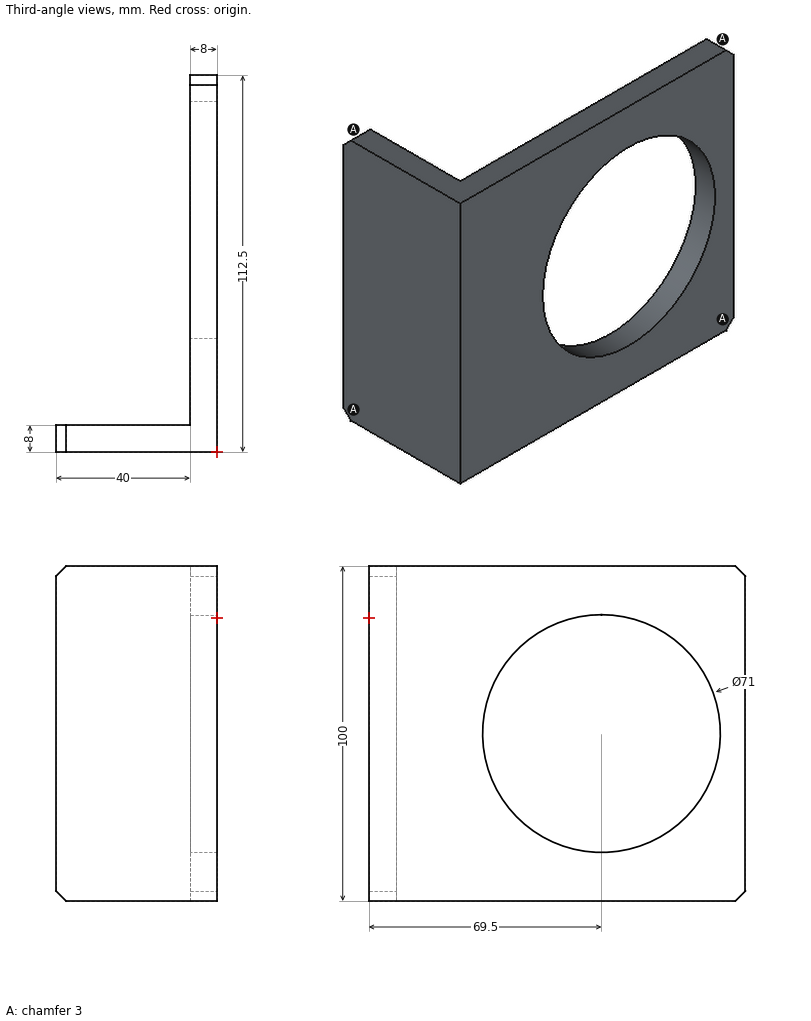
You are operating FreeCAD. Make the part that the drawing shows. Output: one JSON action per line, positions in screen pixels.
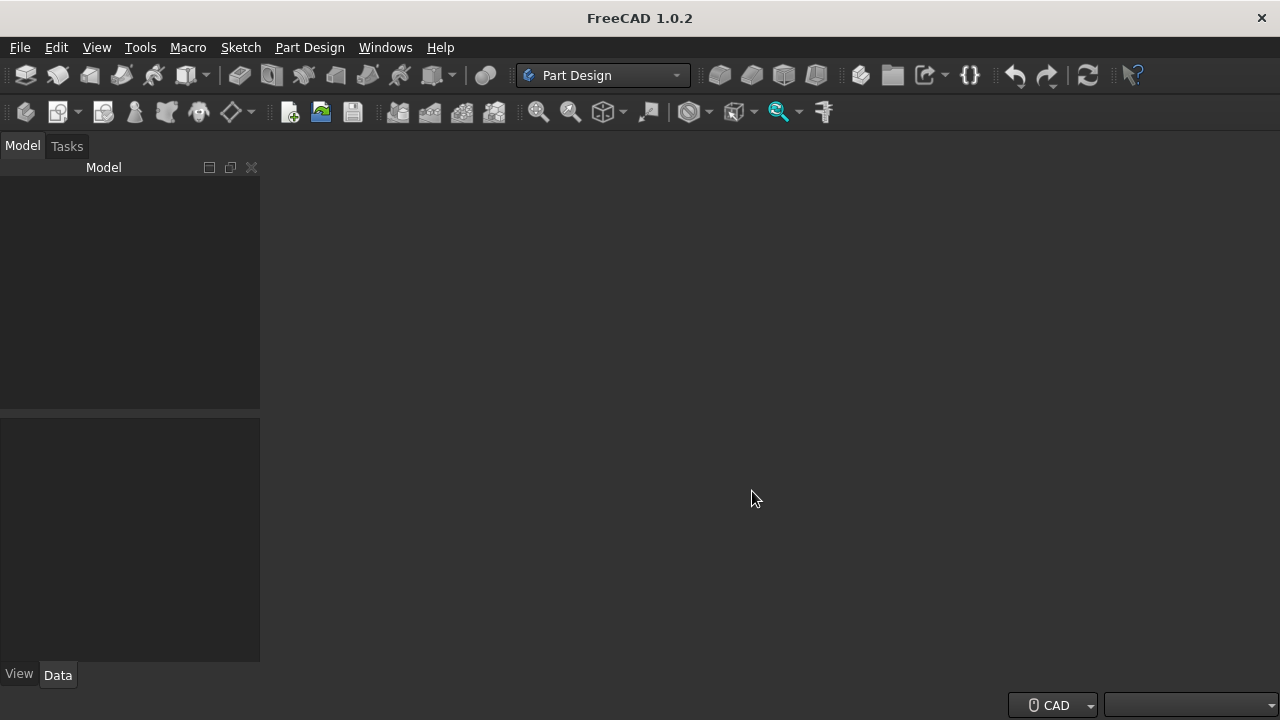
{"action": "left_click", "coordinate": [290, 112]}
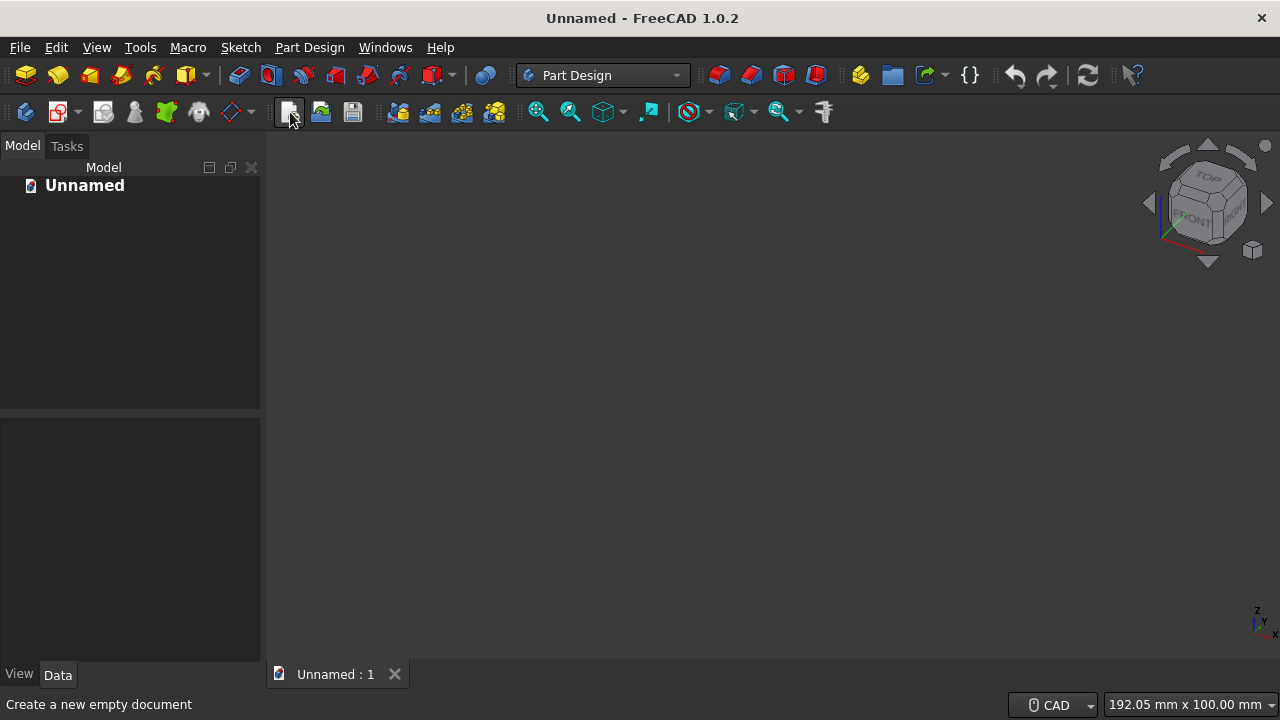
{"action": "left_click", "coordinate": [26, 112]}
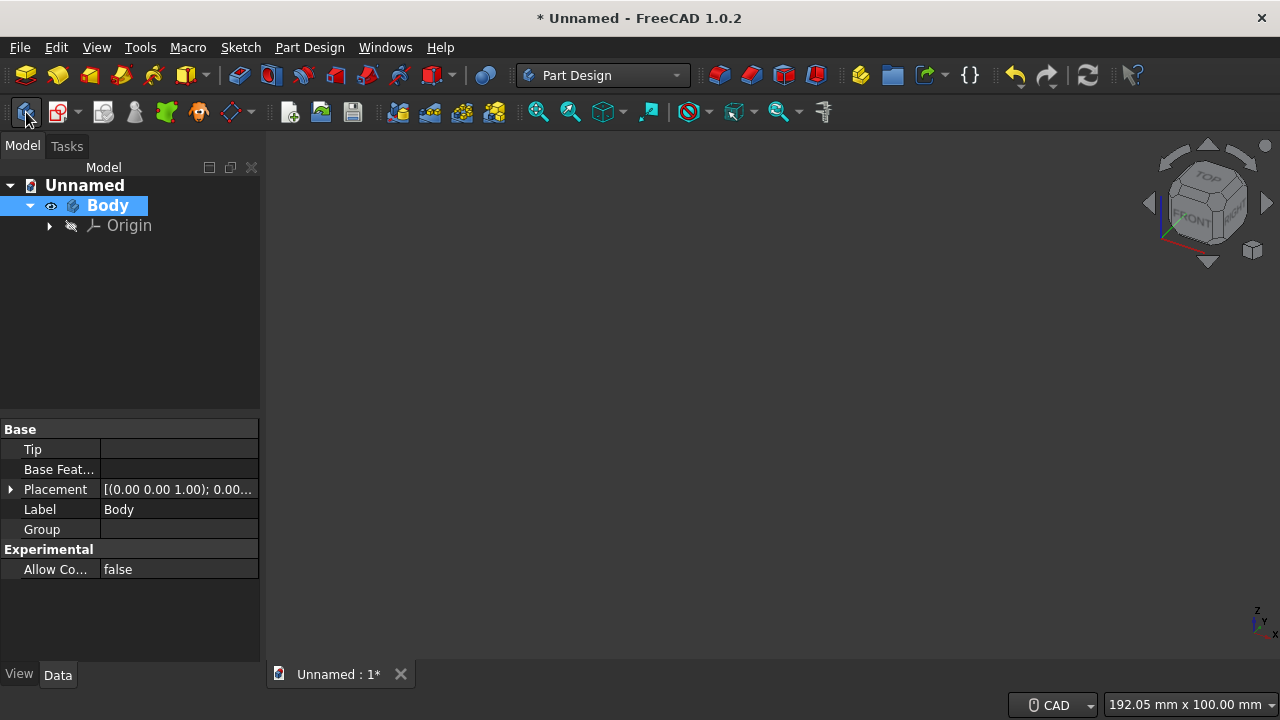
{"action": "left_click", "coordinate": [50, 226]}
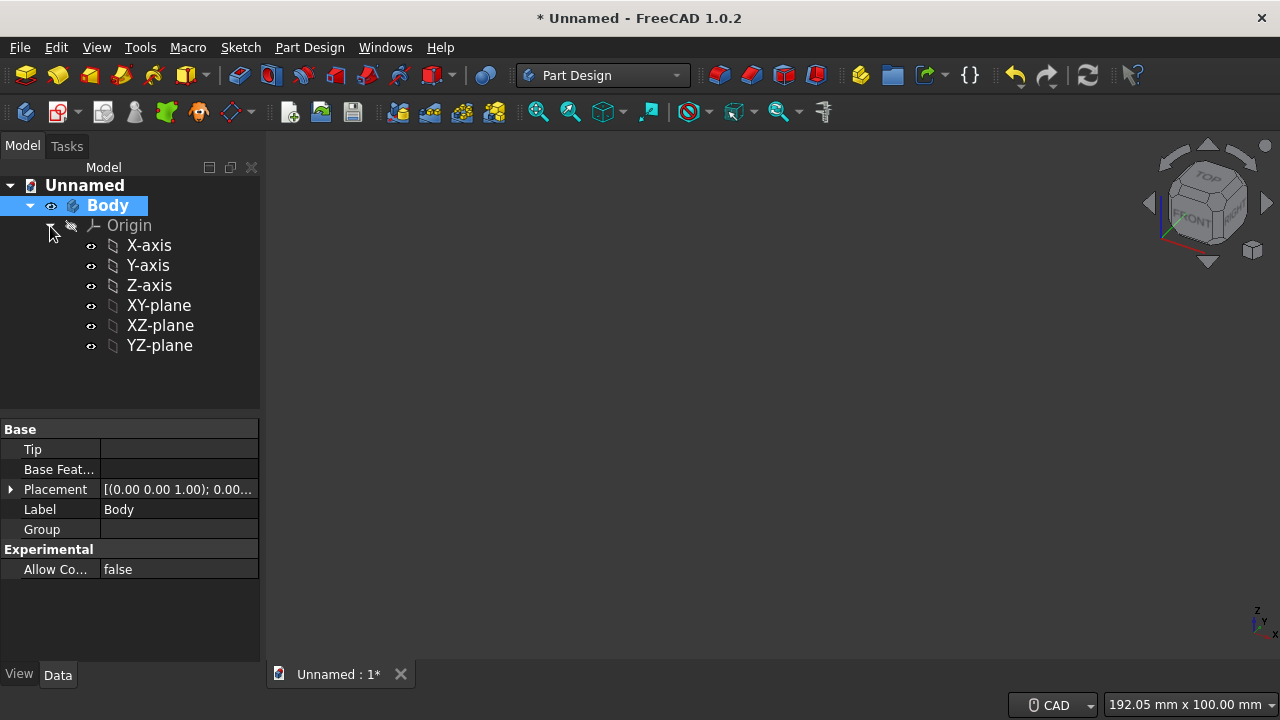
{"action": "left_click", "coordinate": [136, 306]}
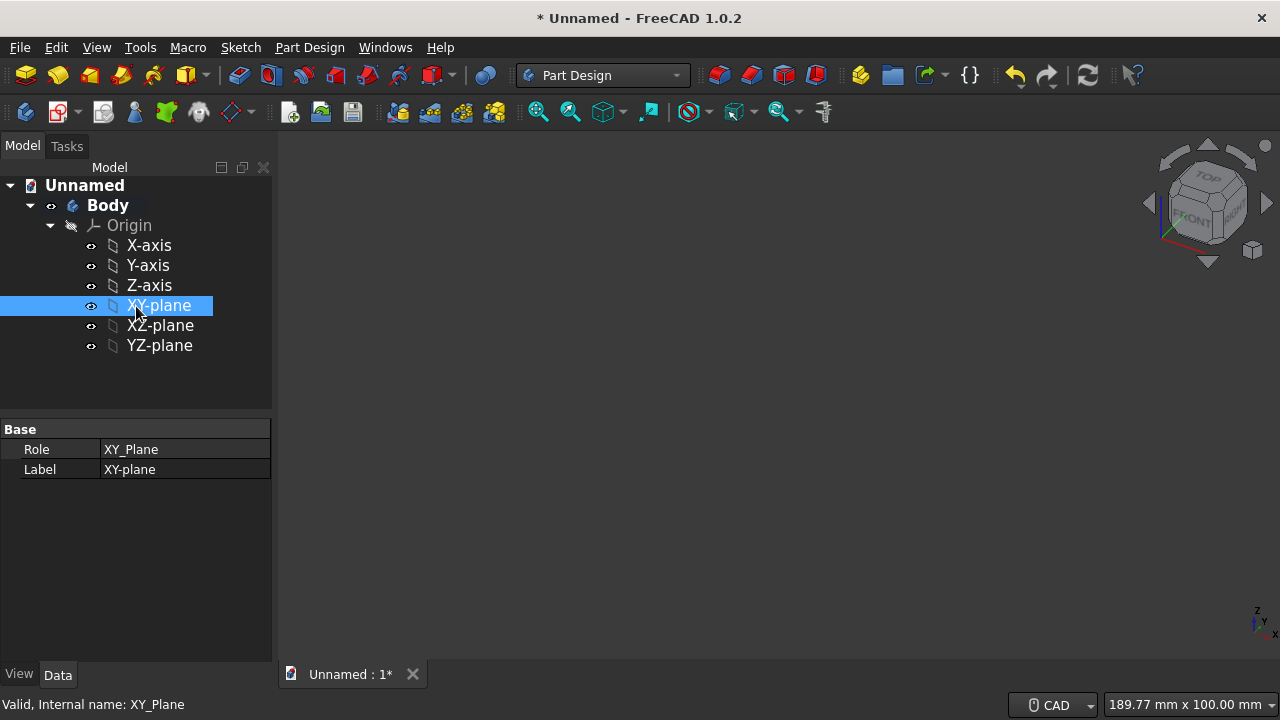
{"action": "left_click", "coordinate": [232, 112]}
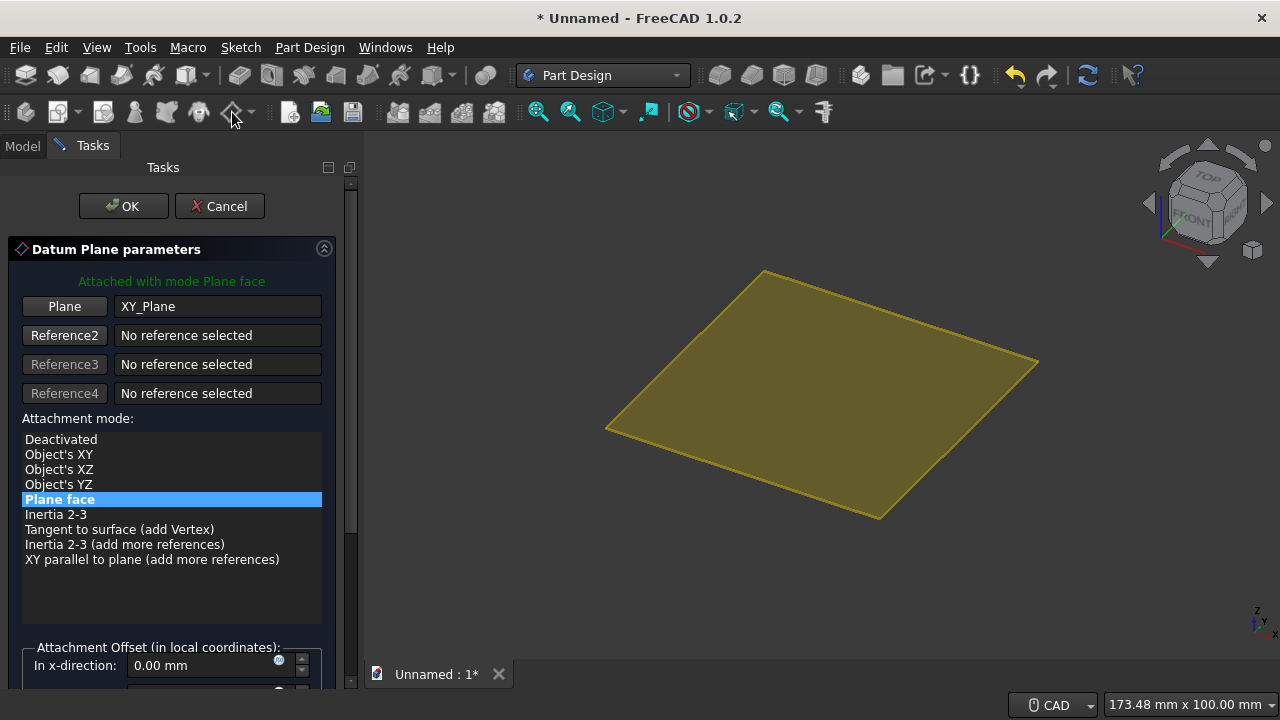
{"action": "scroll", "coordinate": [351, 432], "scroll_direction": "down", "scroll_amount": 2}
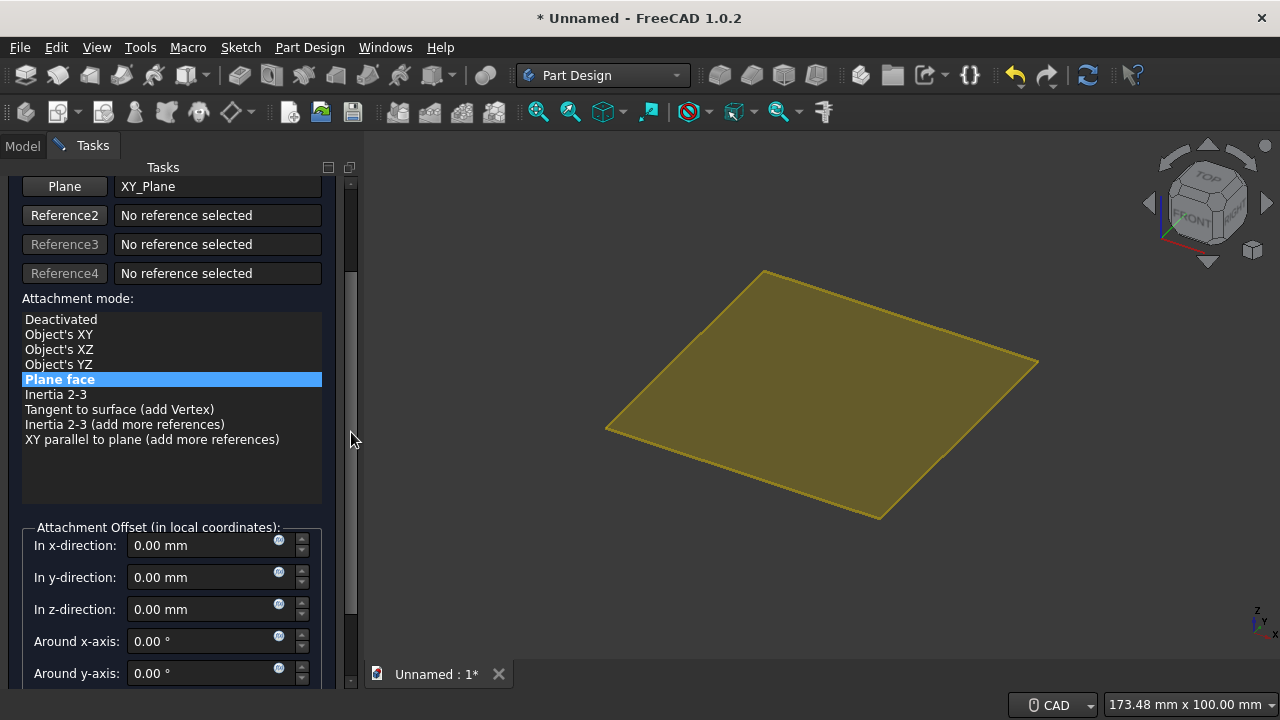
{"action": "triple_click", "coordinate": [210, 609]}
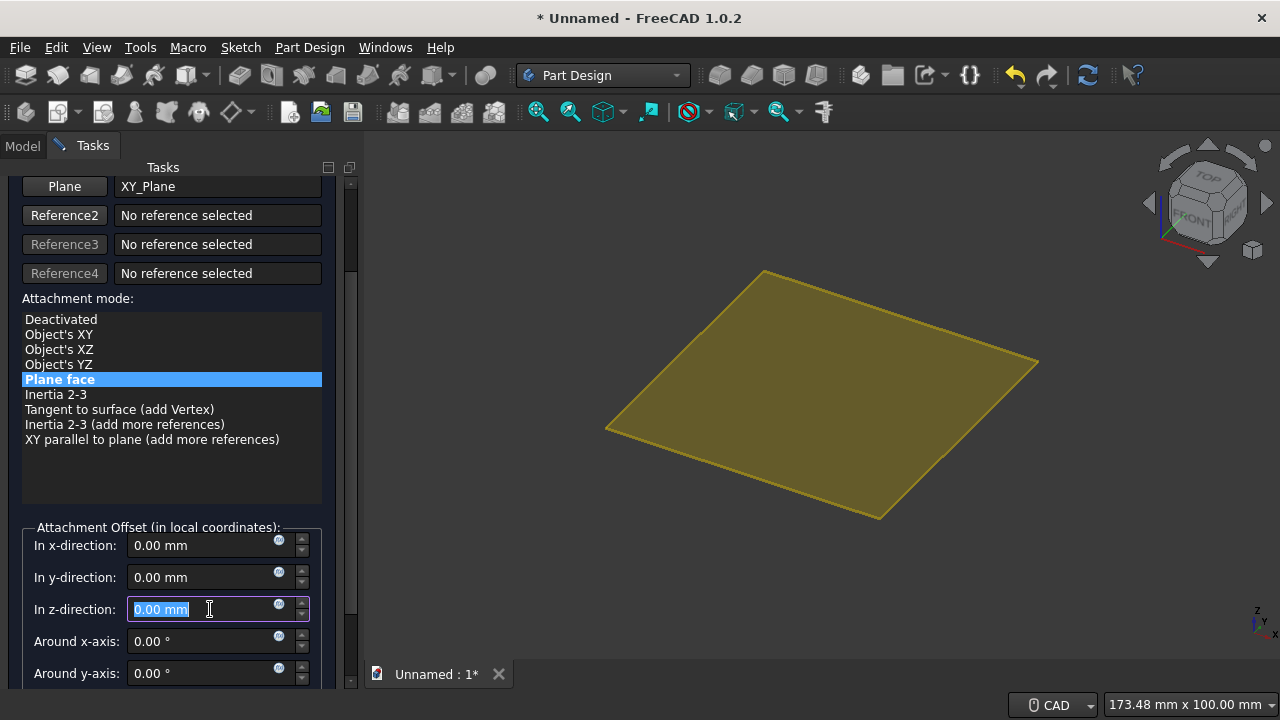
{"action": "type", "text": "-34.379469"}
{"action": "key", "text": "Tab"}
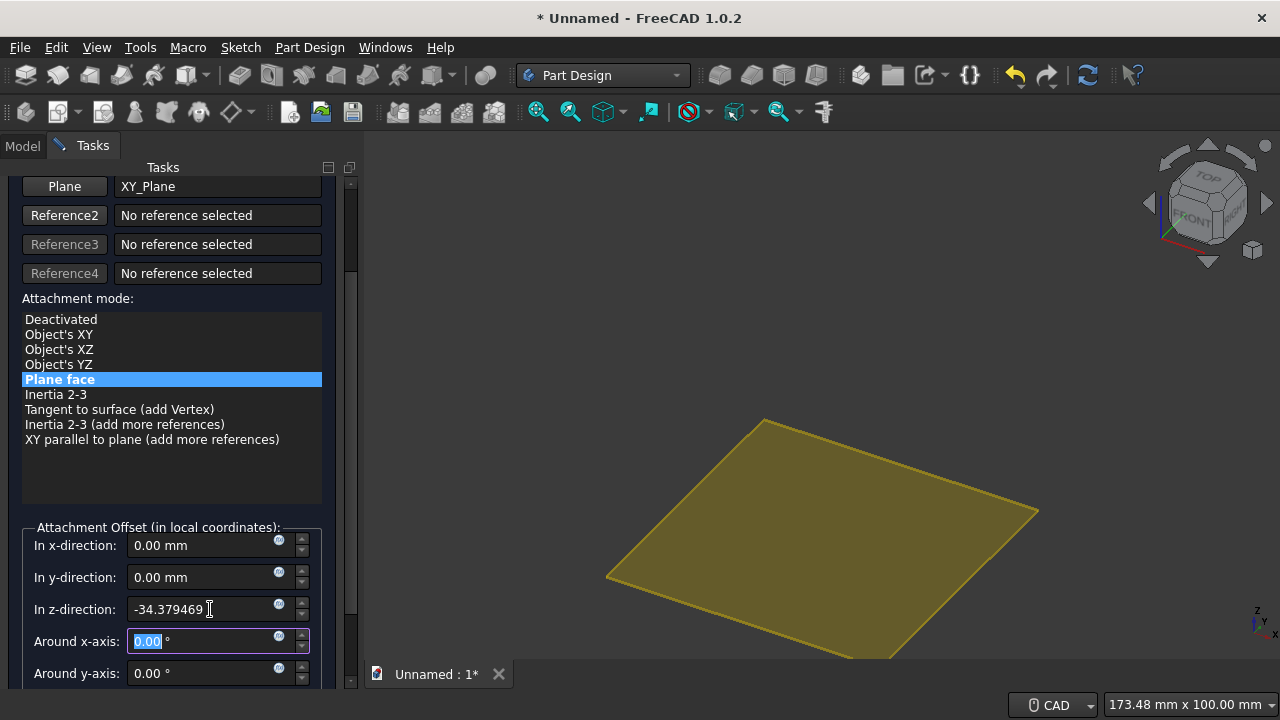
{"action": "scroll", "coordinate": [351, 432], "scroll_direction": "up", "scroll_amount": 3}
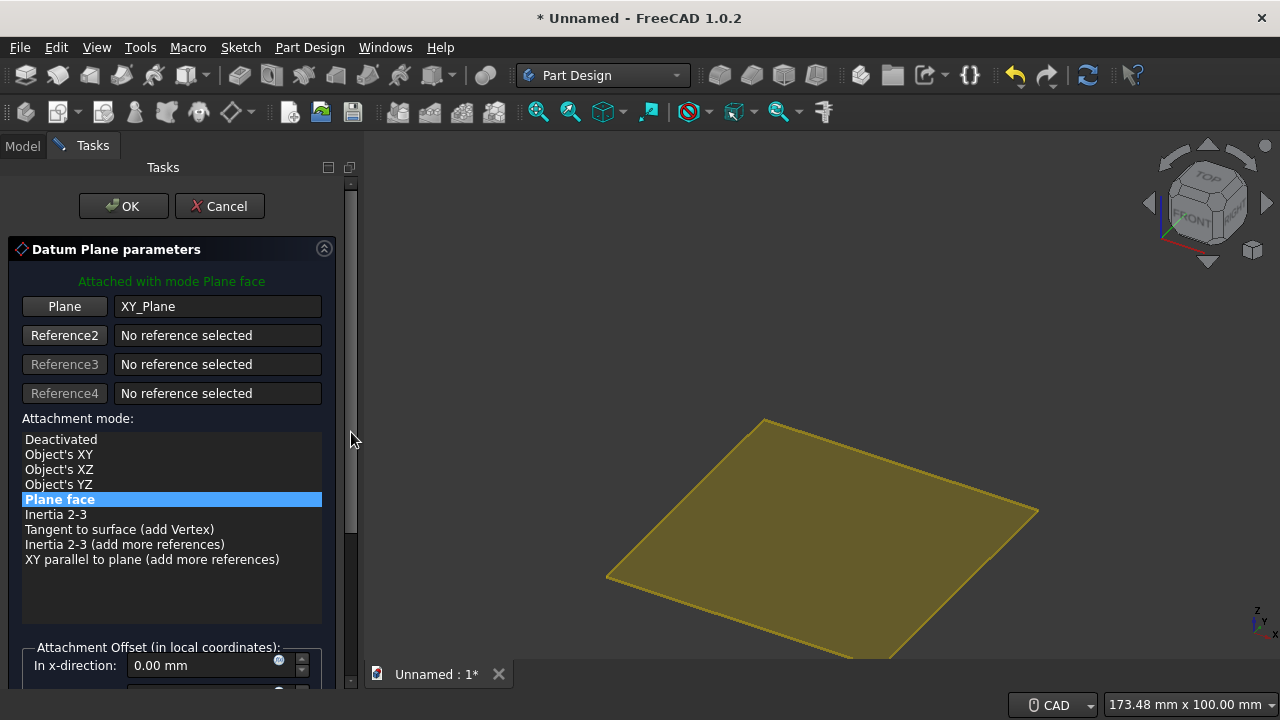
{"action": "left_click", "coordinate": [124, 206]}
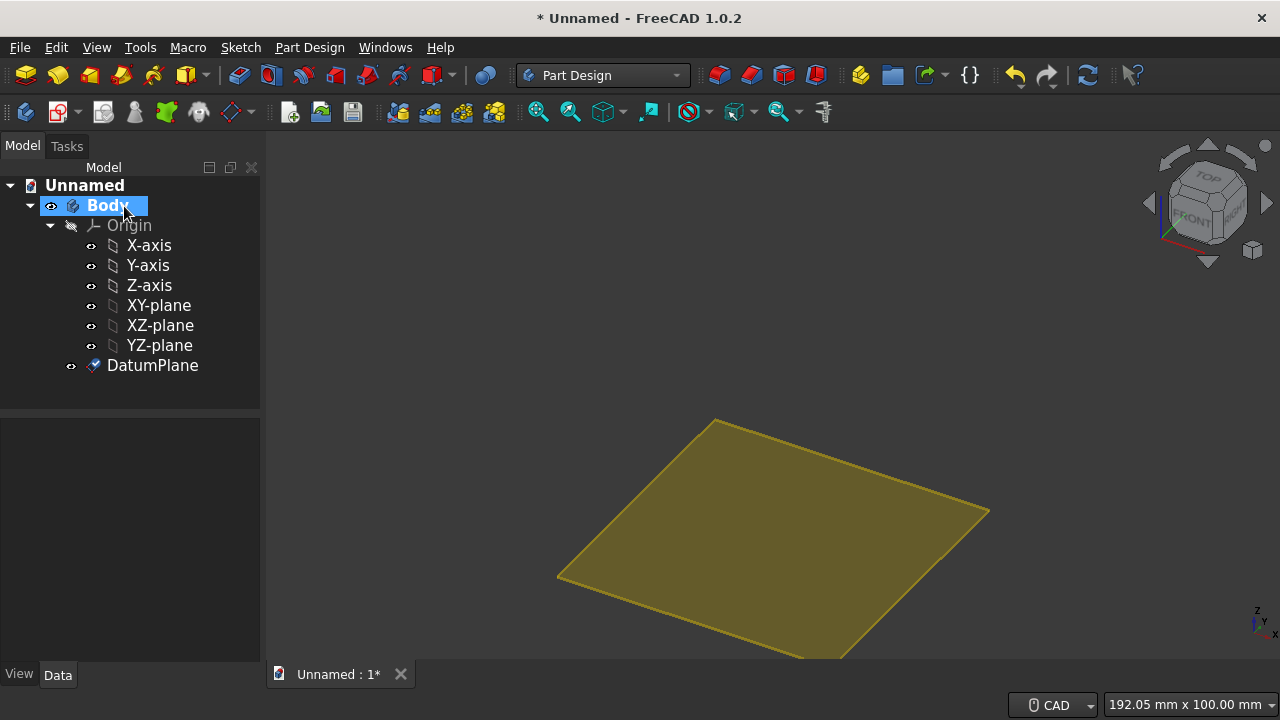
{"action": "left_click", "coordinate": [116, 366]}